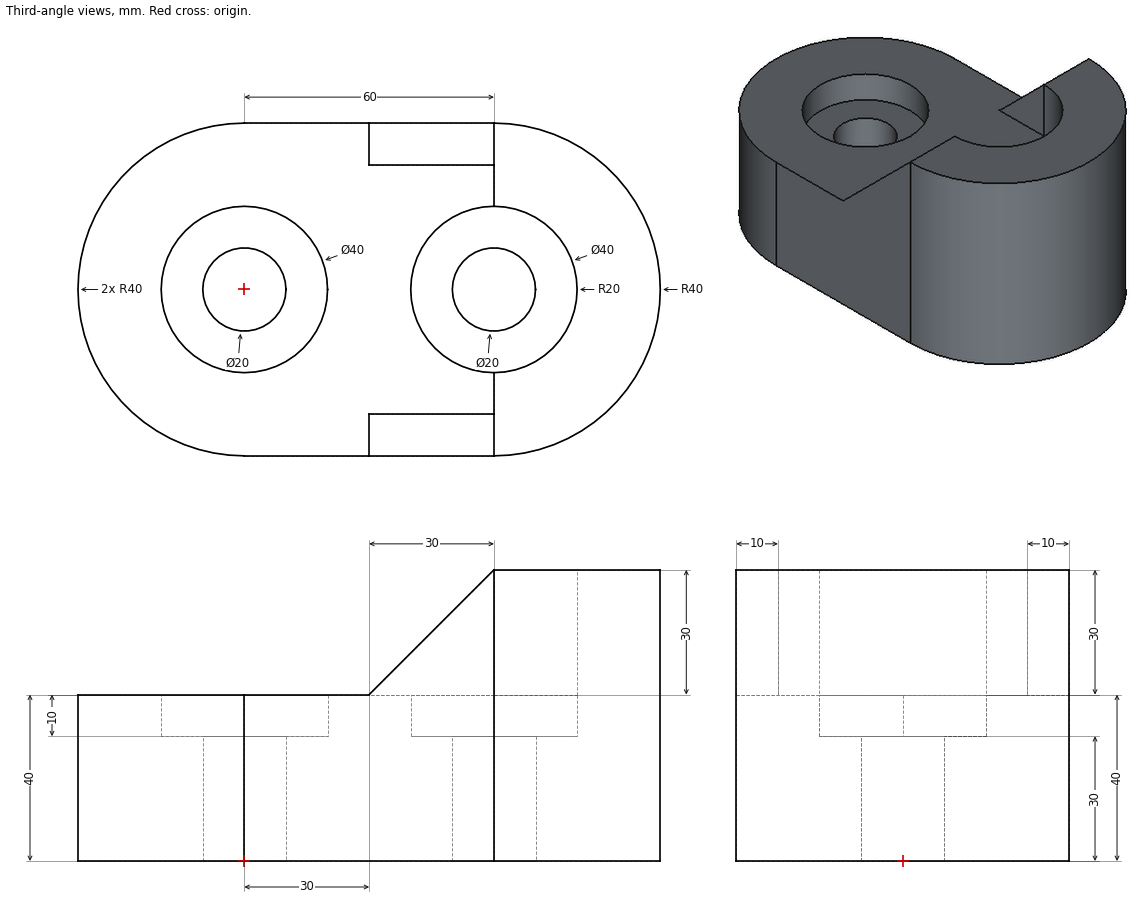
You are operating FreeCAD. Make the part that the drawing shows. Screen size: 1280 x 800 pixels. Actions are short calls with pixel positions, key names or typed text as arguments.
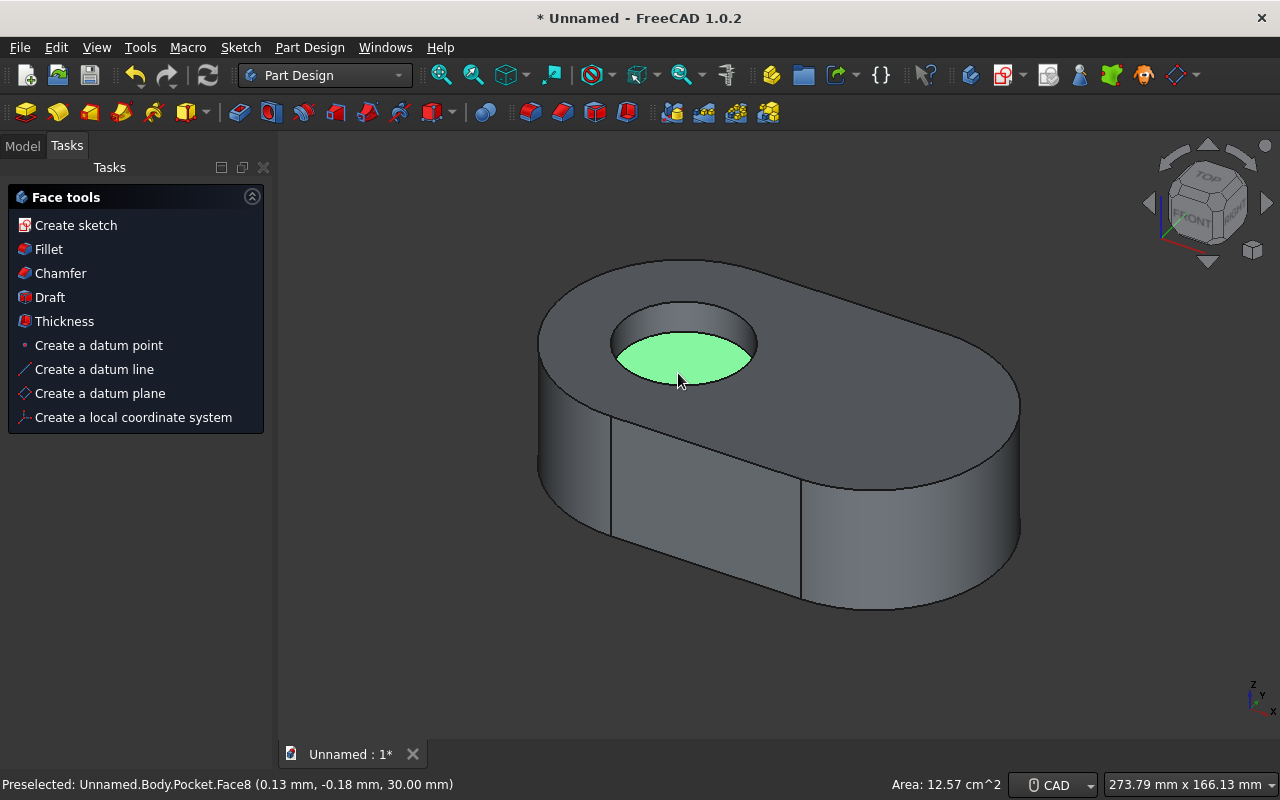
click(1004, 76)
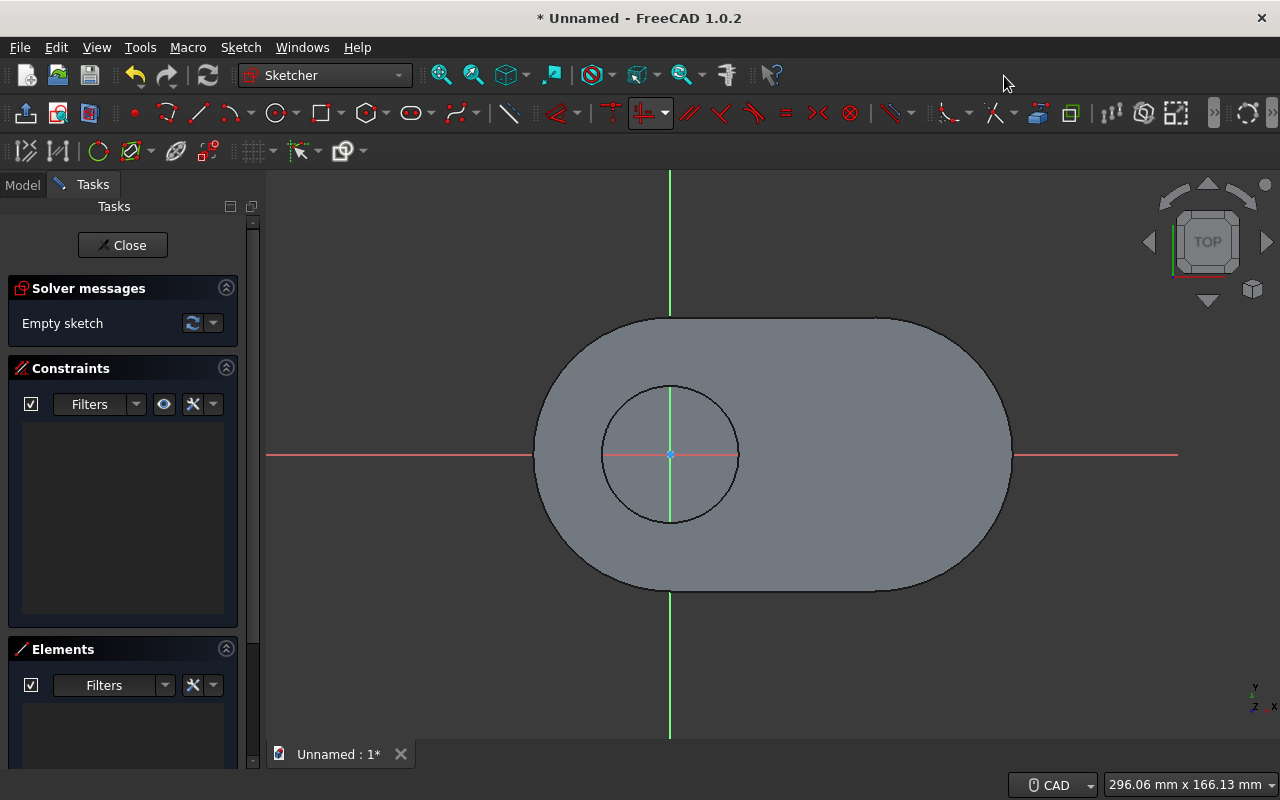
click(90, 114)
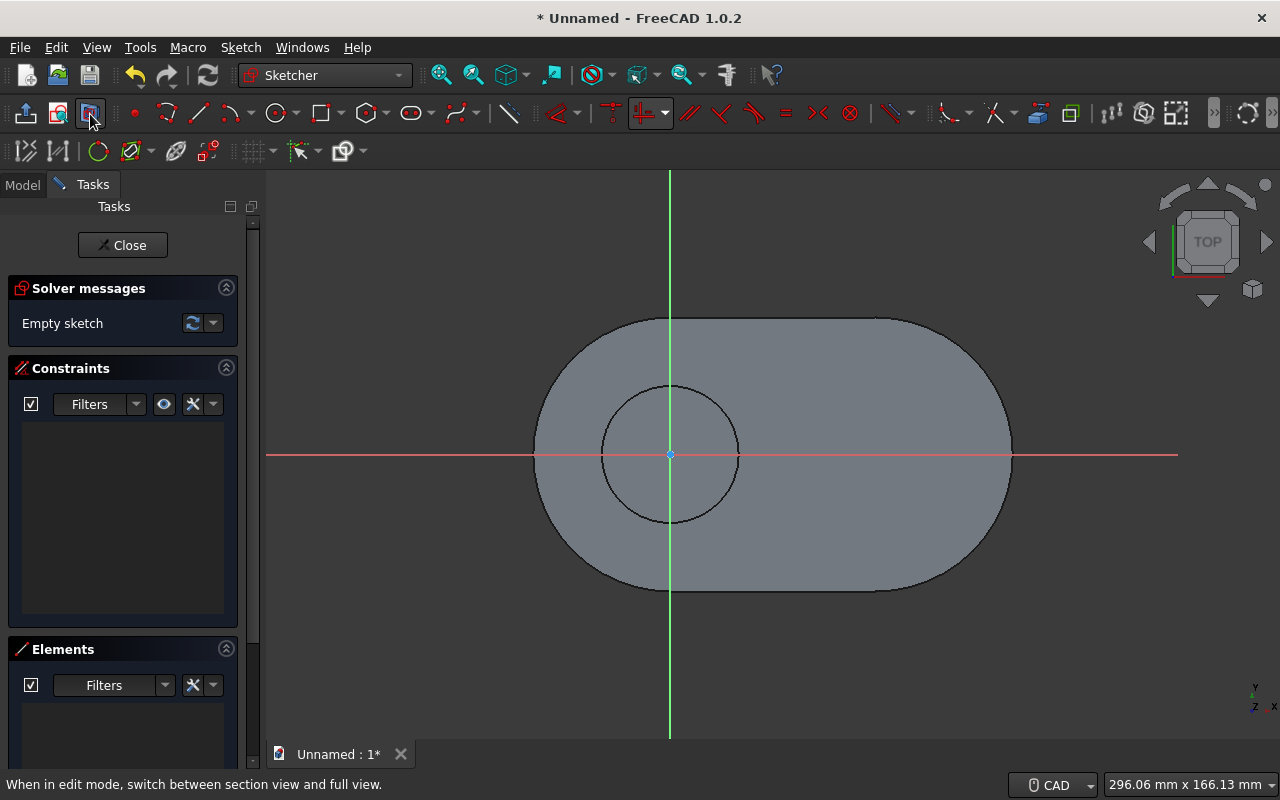
scroll(662, 455, up, 8)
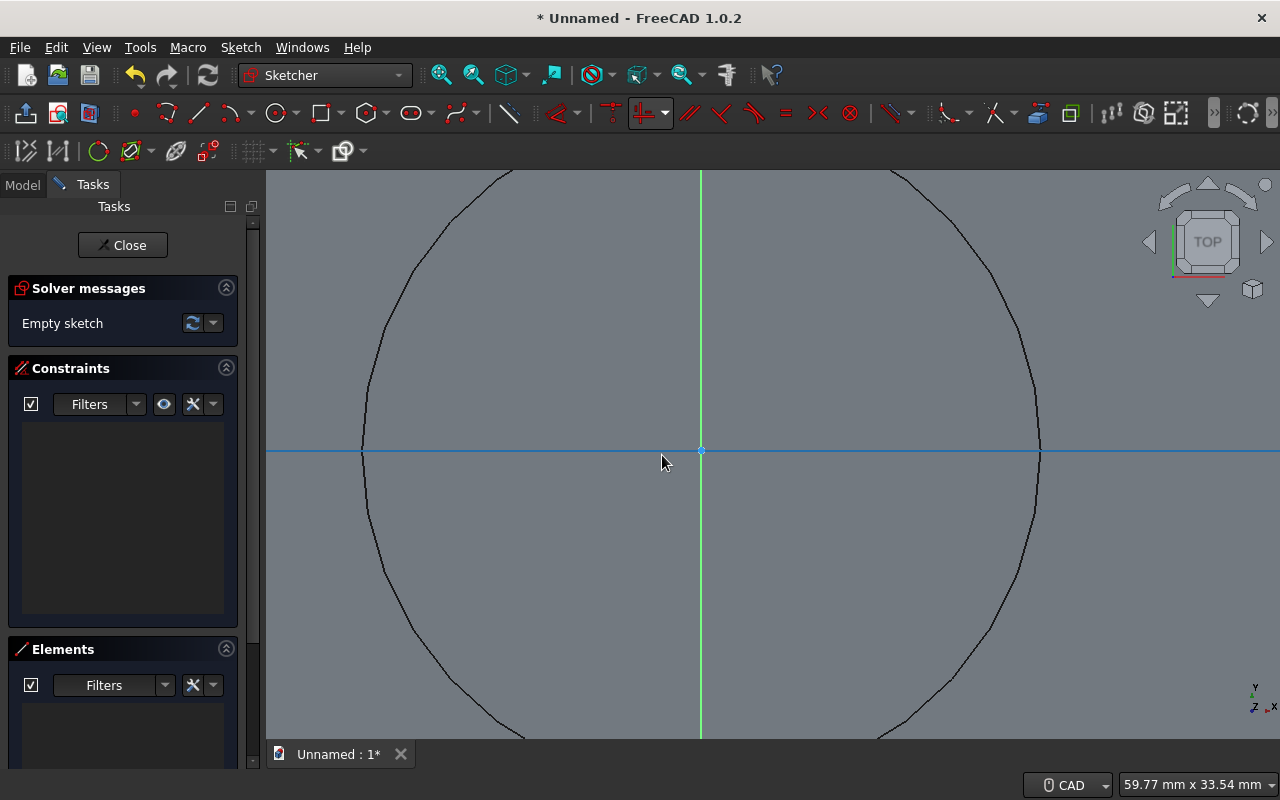
click(276, 114)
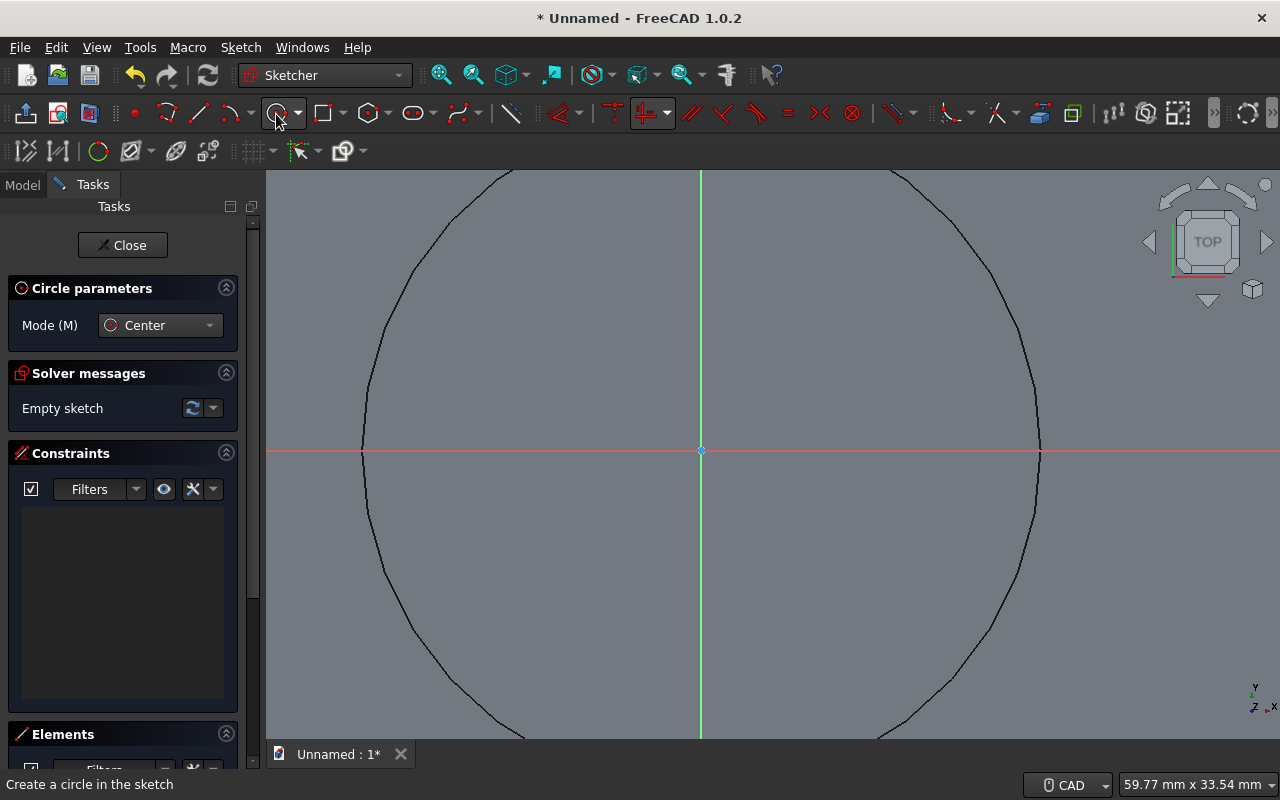
click(701, 451)
move(821, 331)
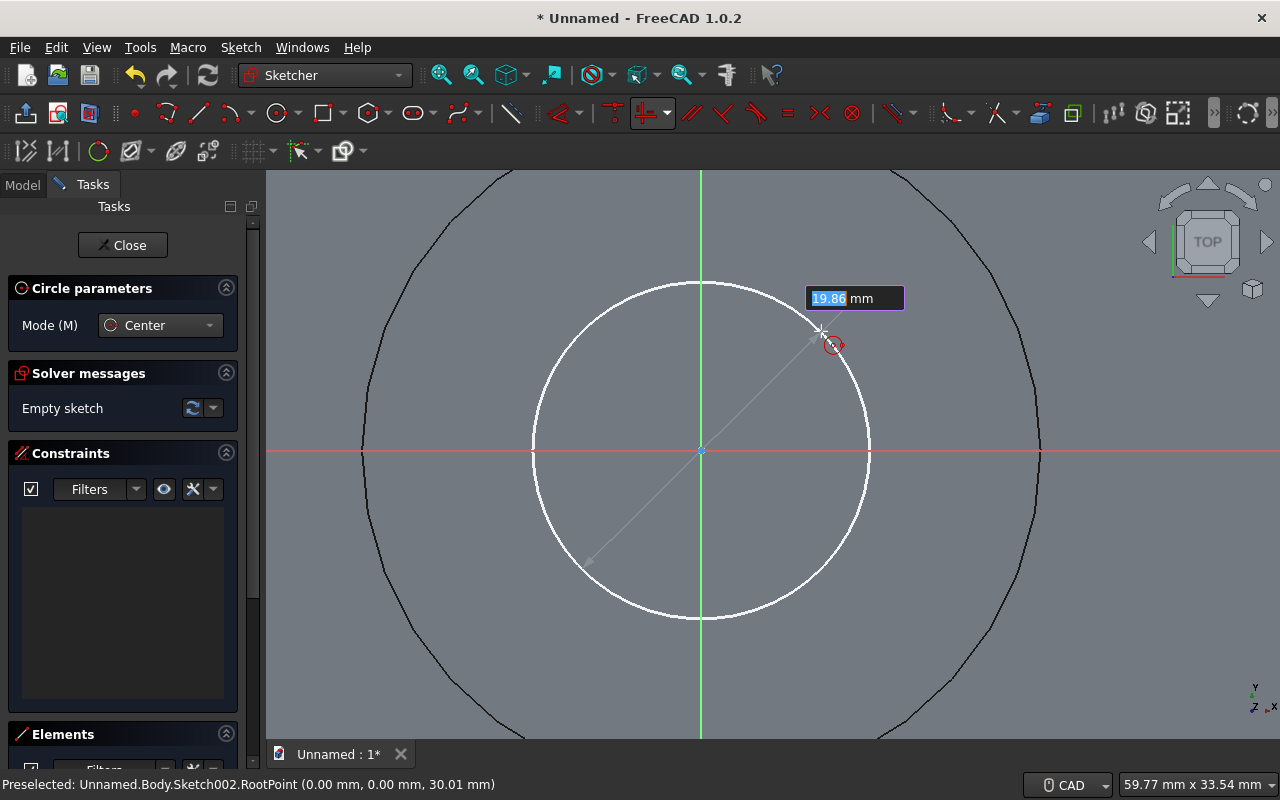
text(20)
key(Return)
key(Escape)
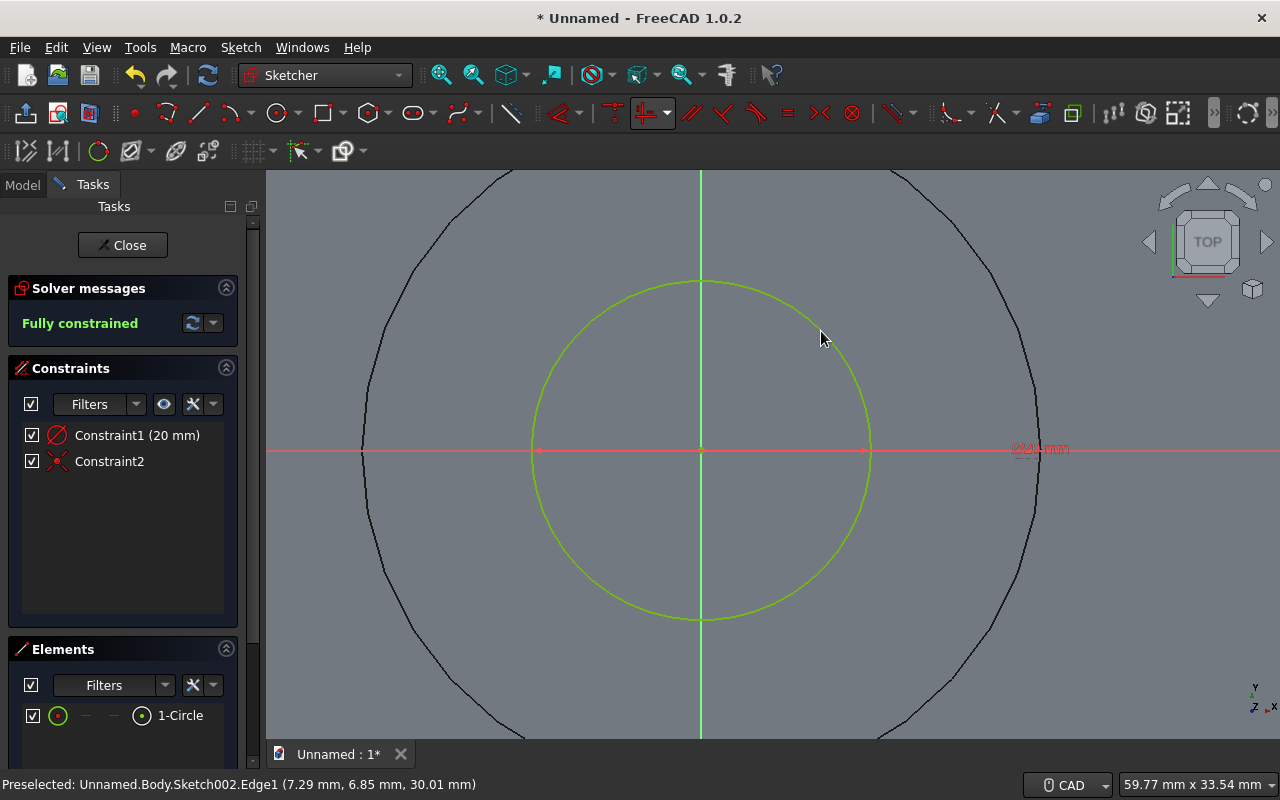
click(123, 245)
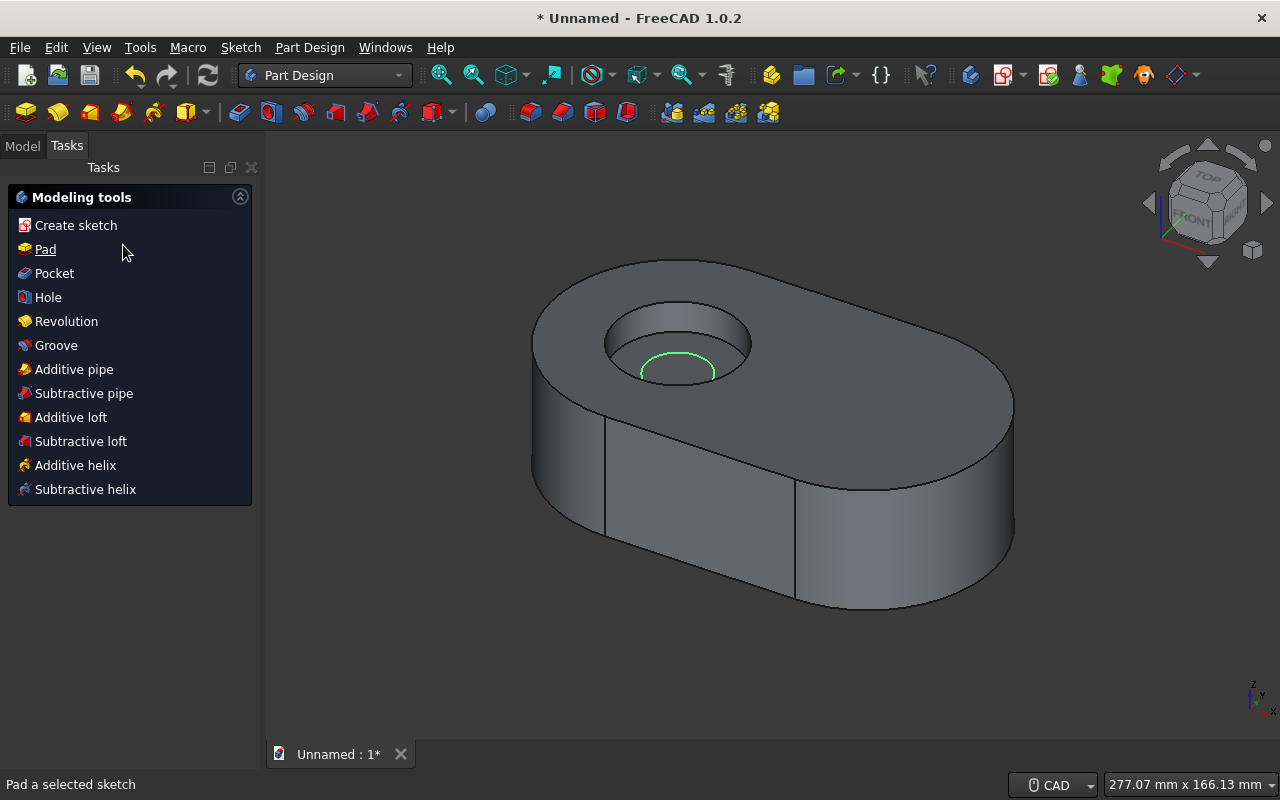
click(240, 112)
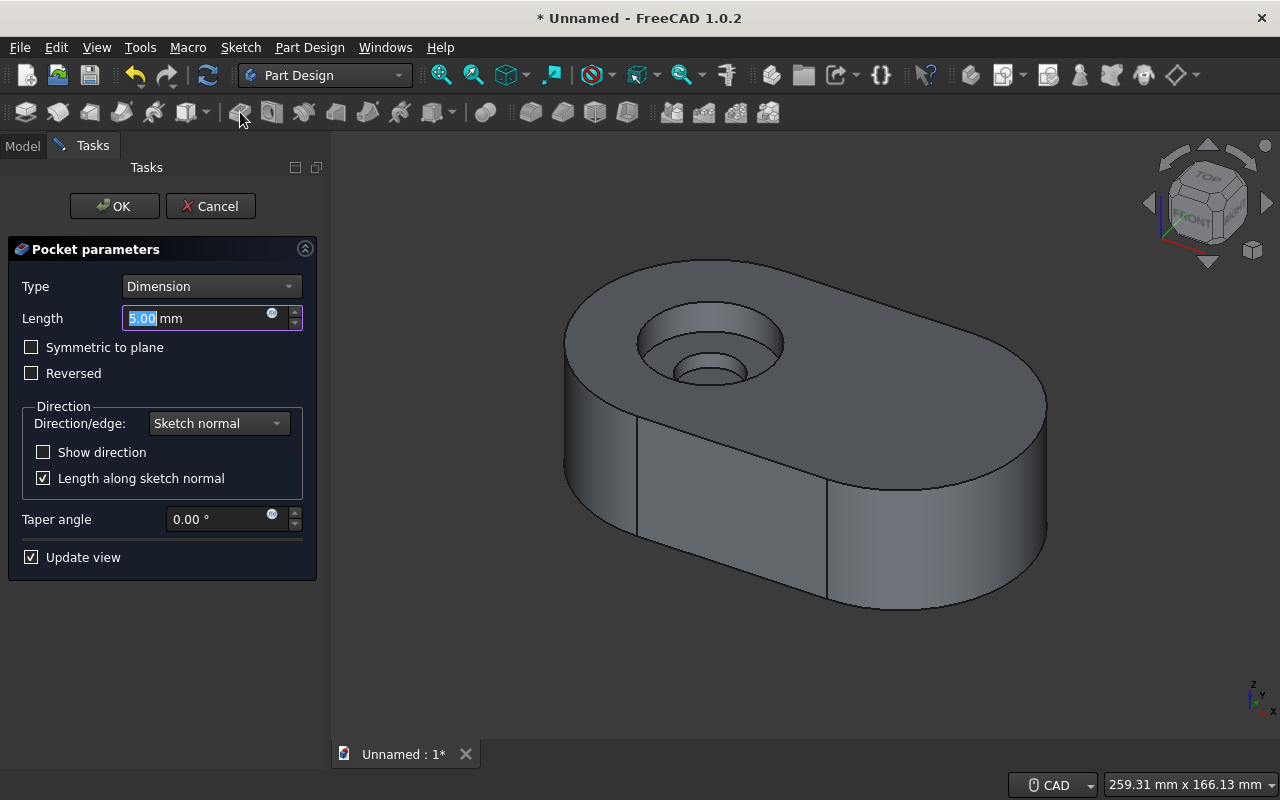
text(30)
key(Tab)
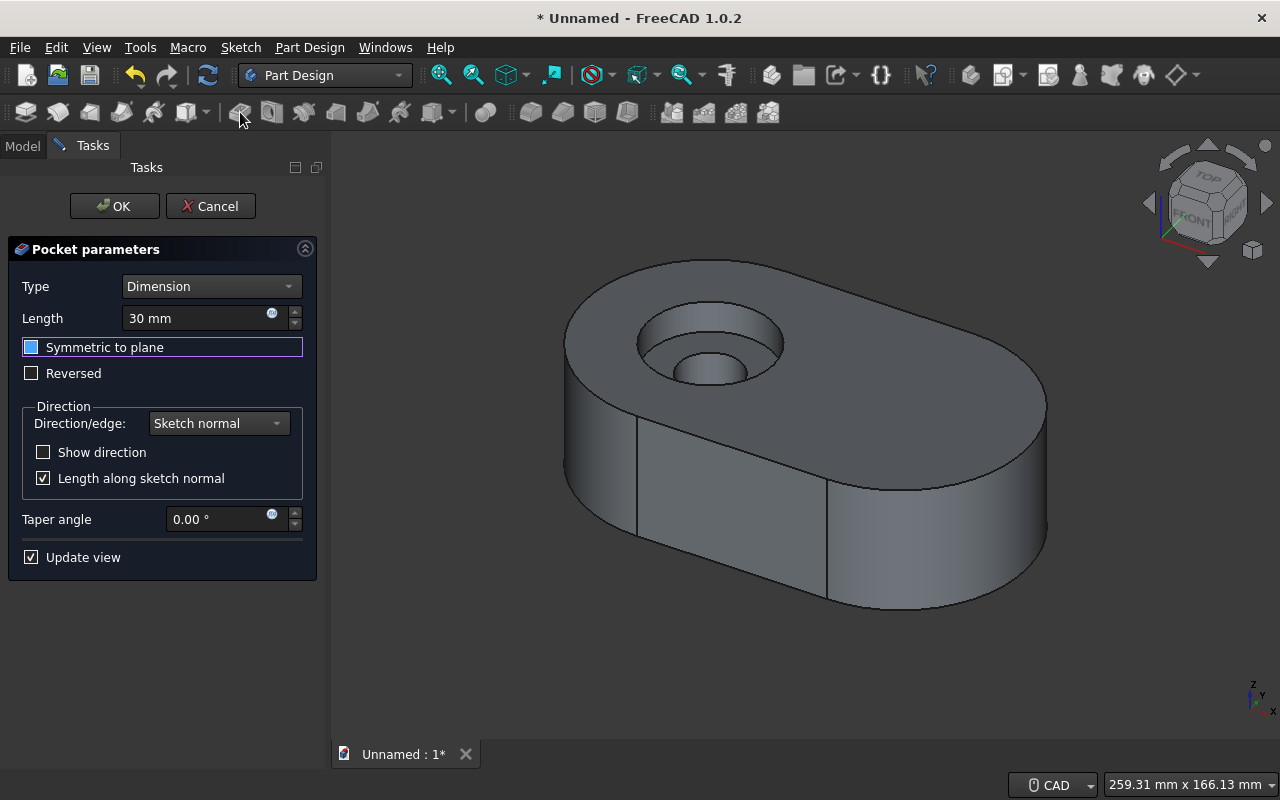
click(115, 206)